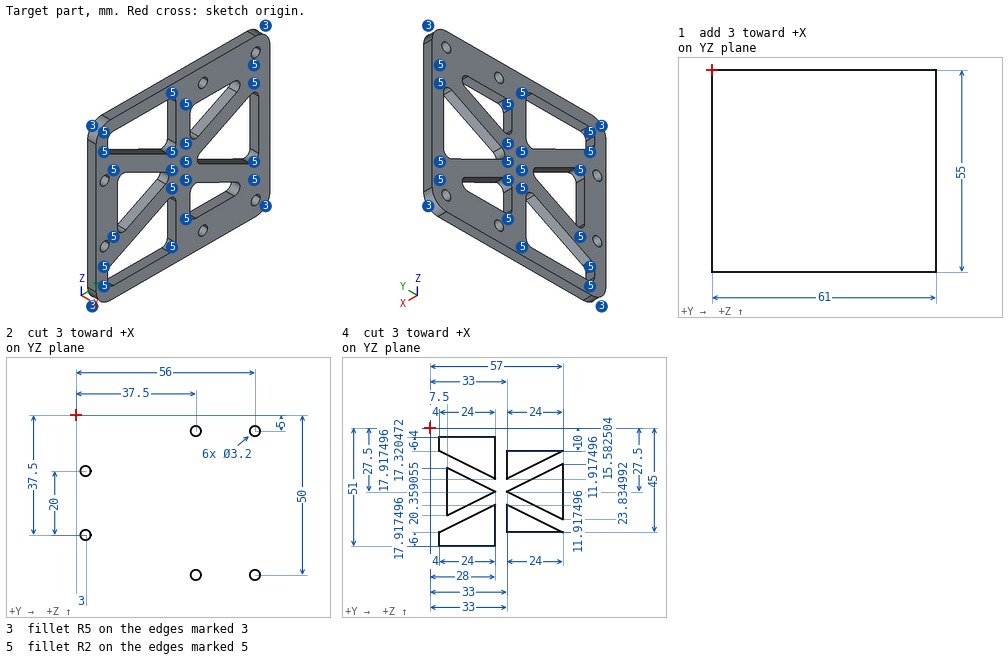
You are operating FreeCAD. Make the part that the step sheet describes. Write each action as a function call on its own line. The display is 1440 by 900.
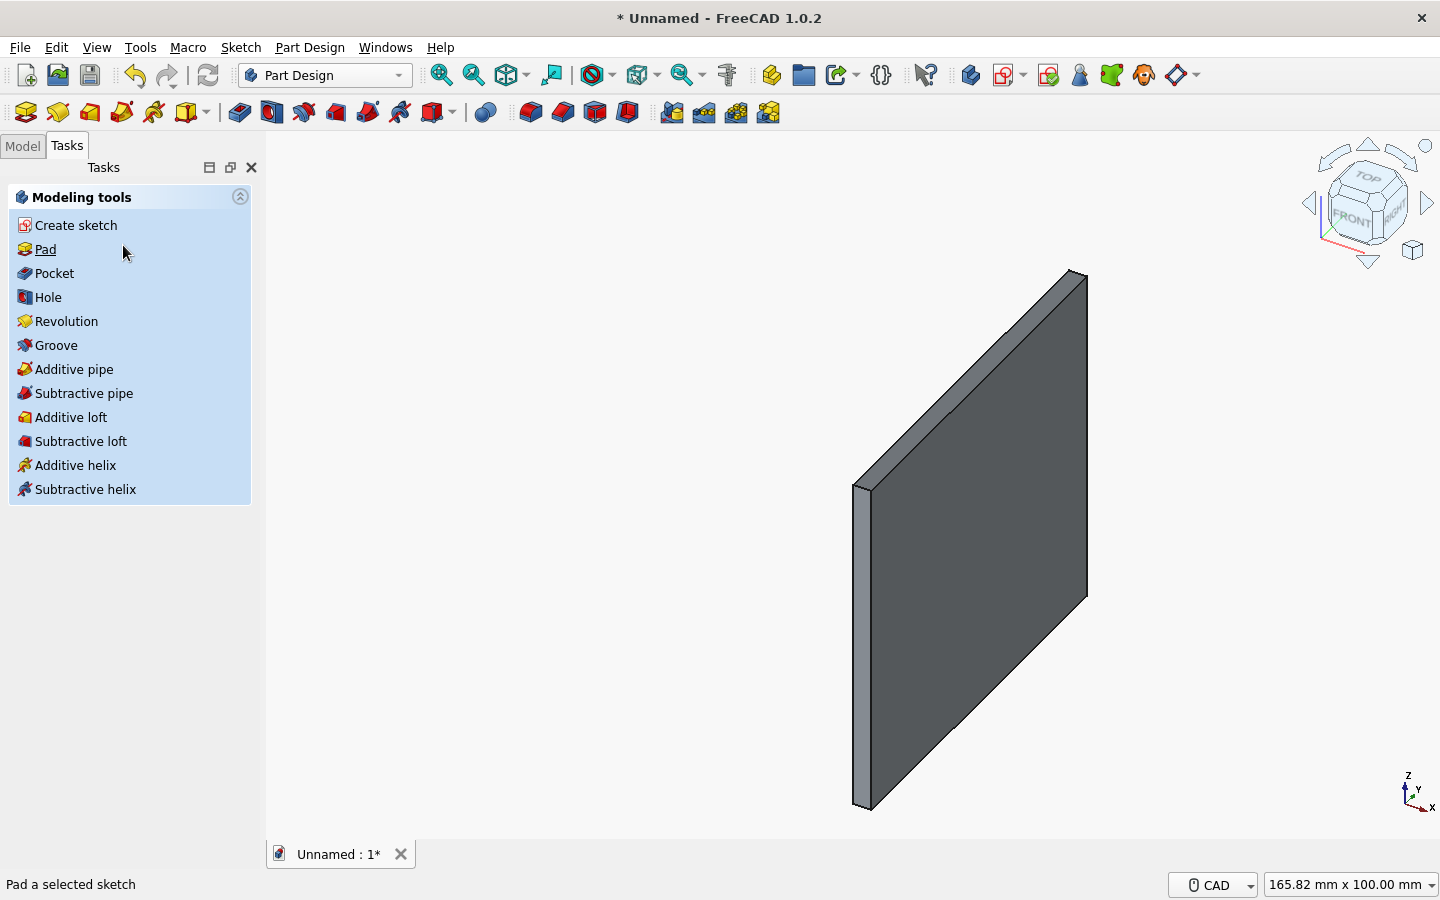
click(240, 112)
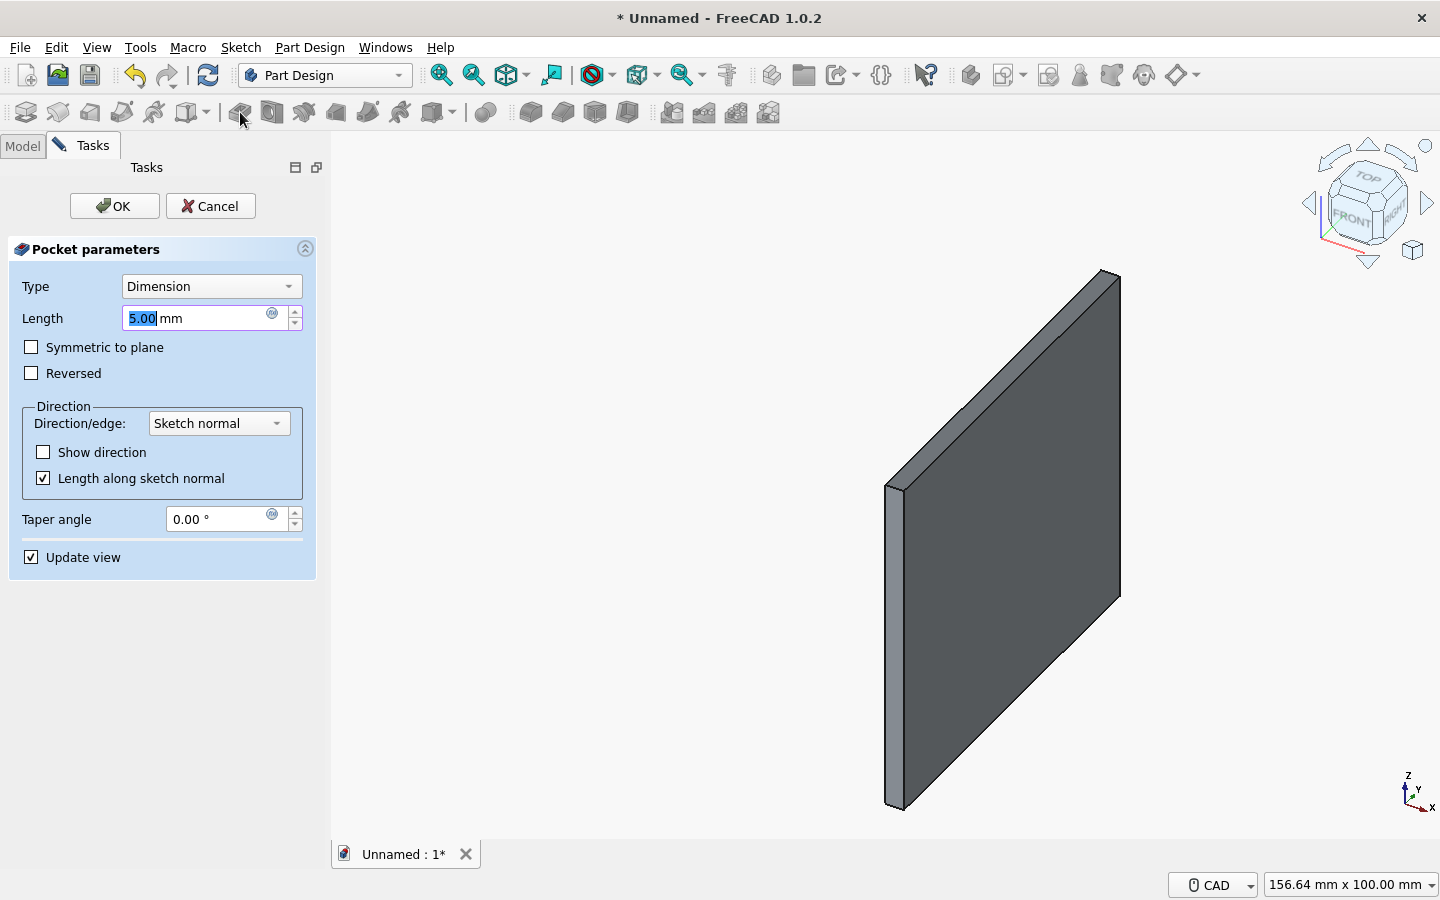
text(3)
key(Tab)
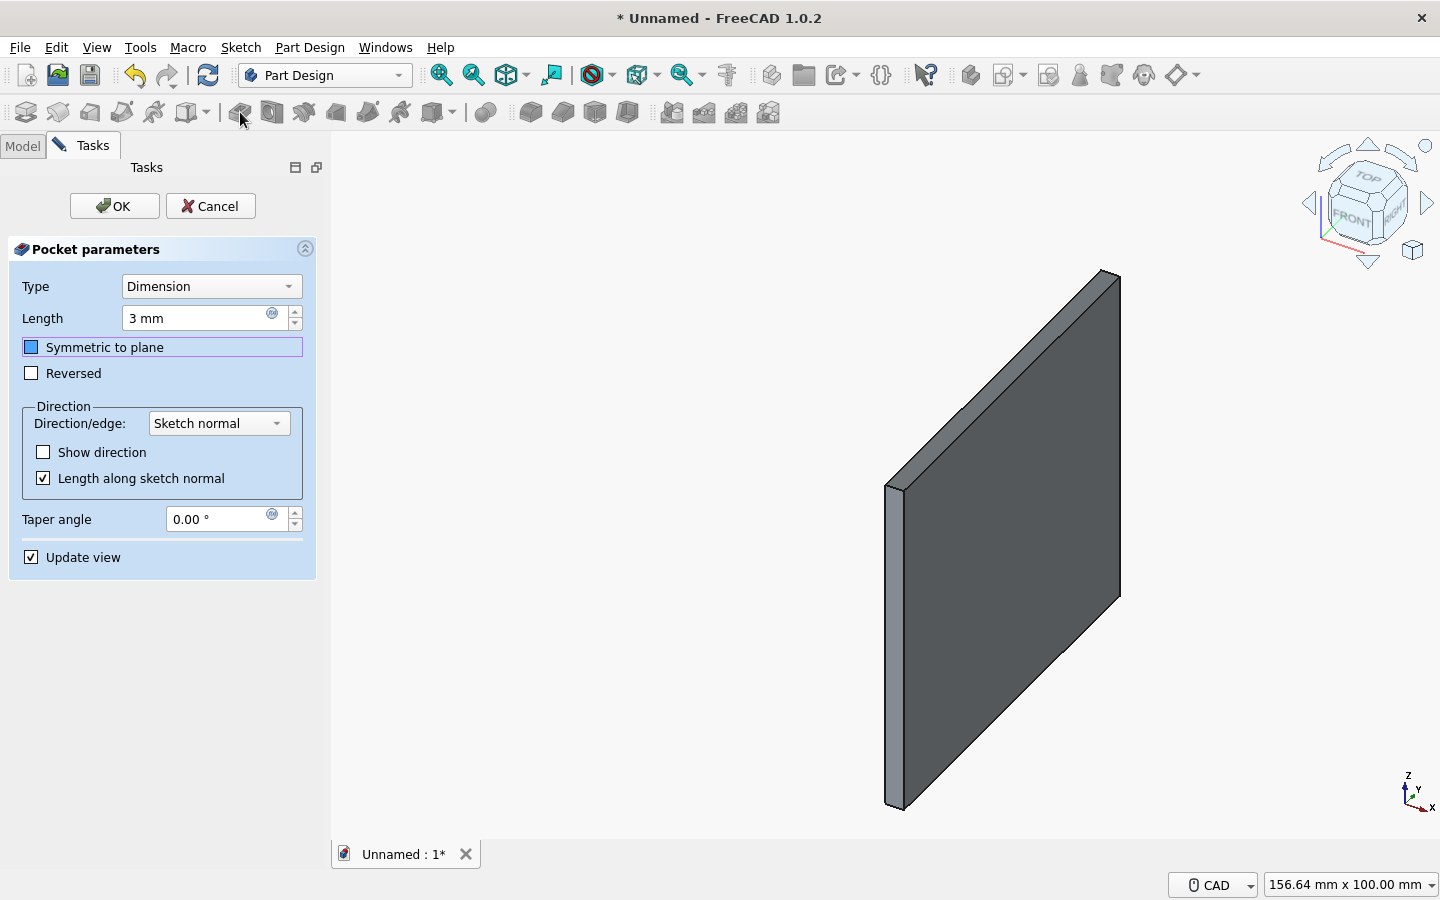
click(30, 373)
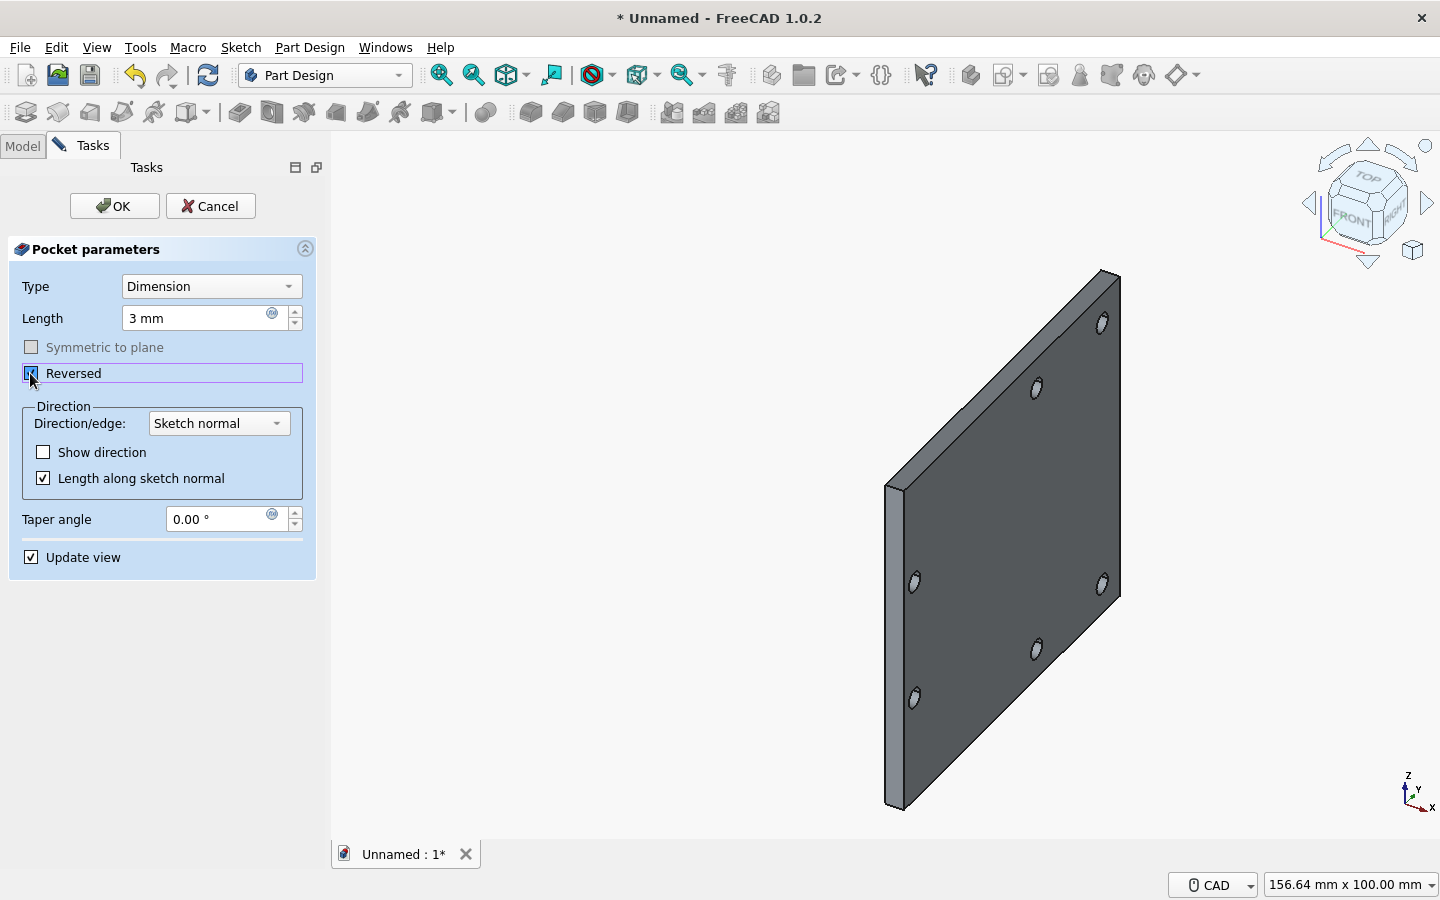
click(115, 206)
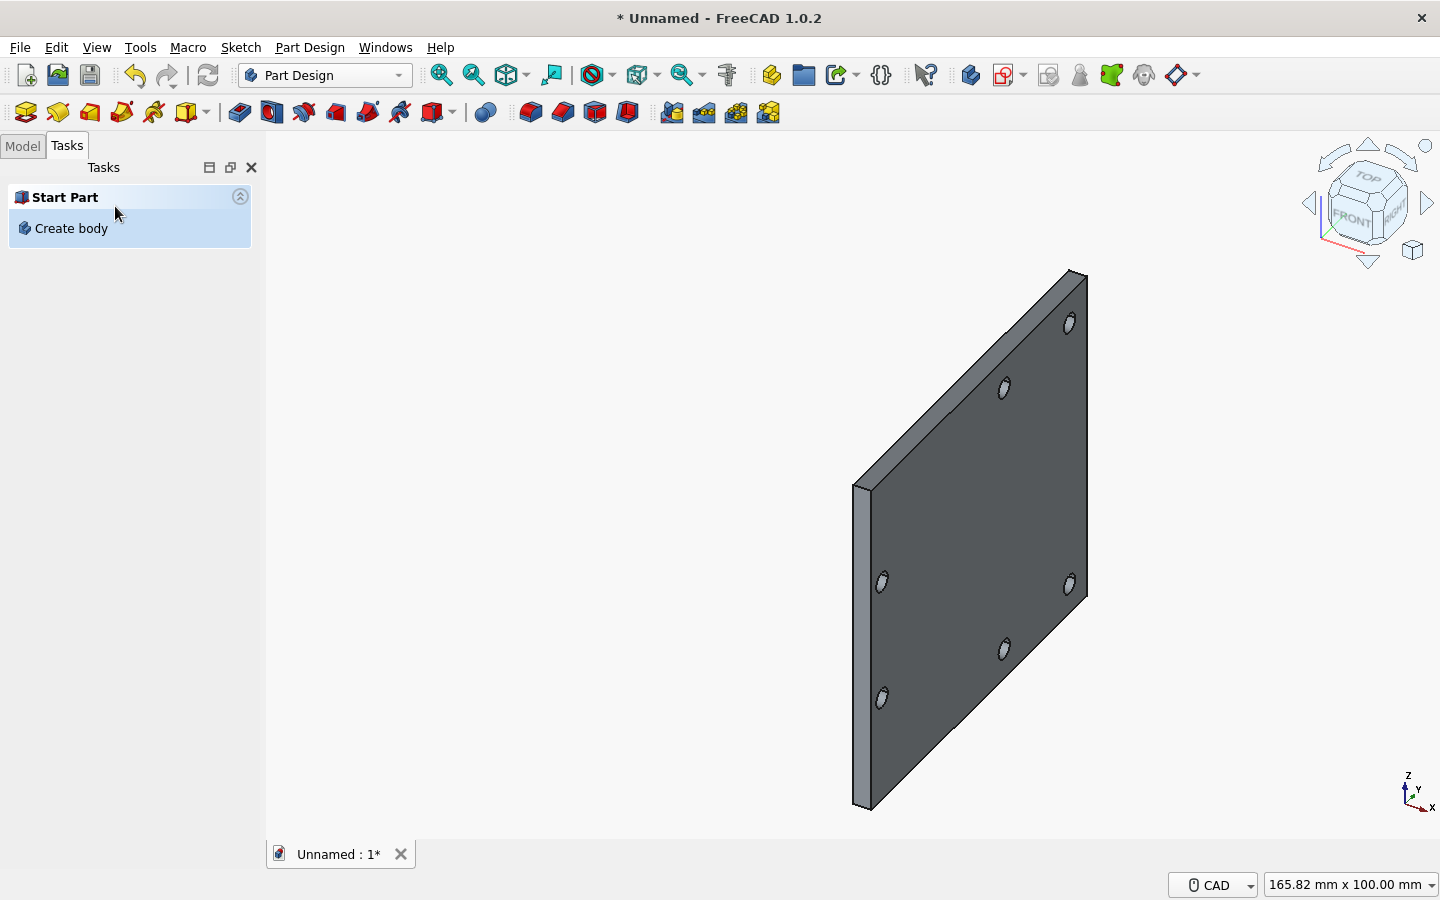
click(862, 487)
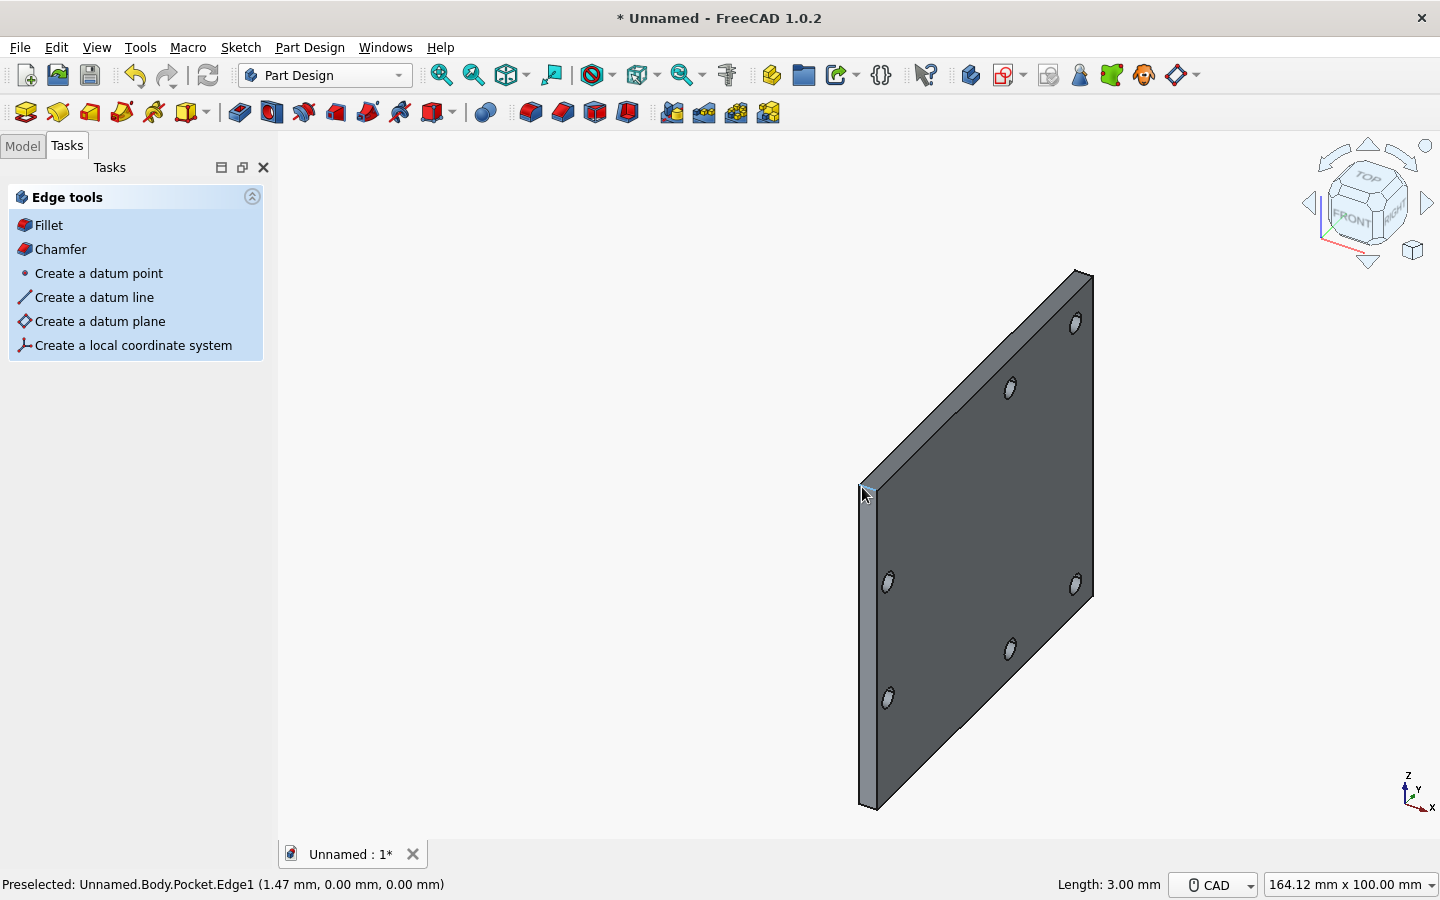
scroll(1084, 273, up, 4)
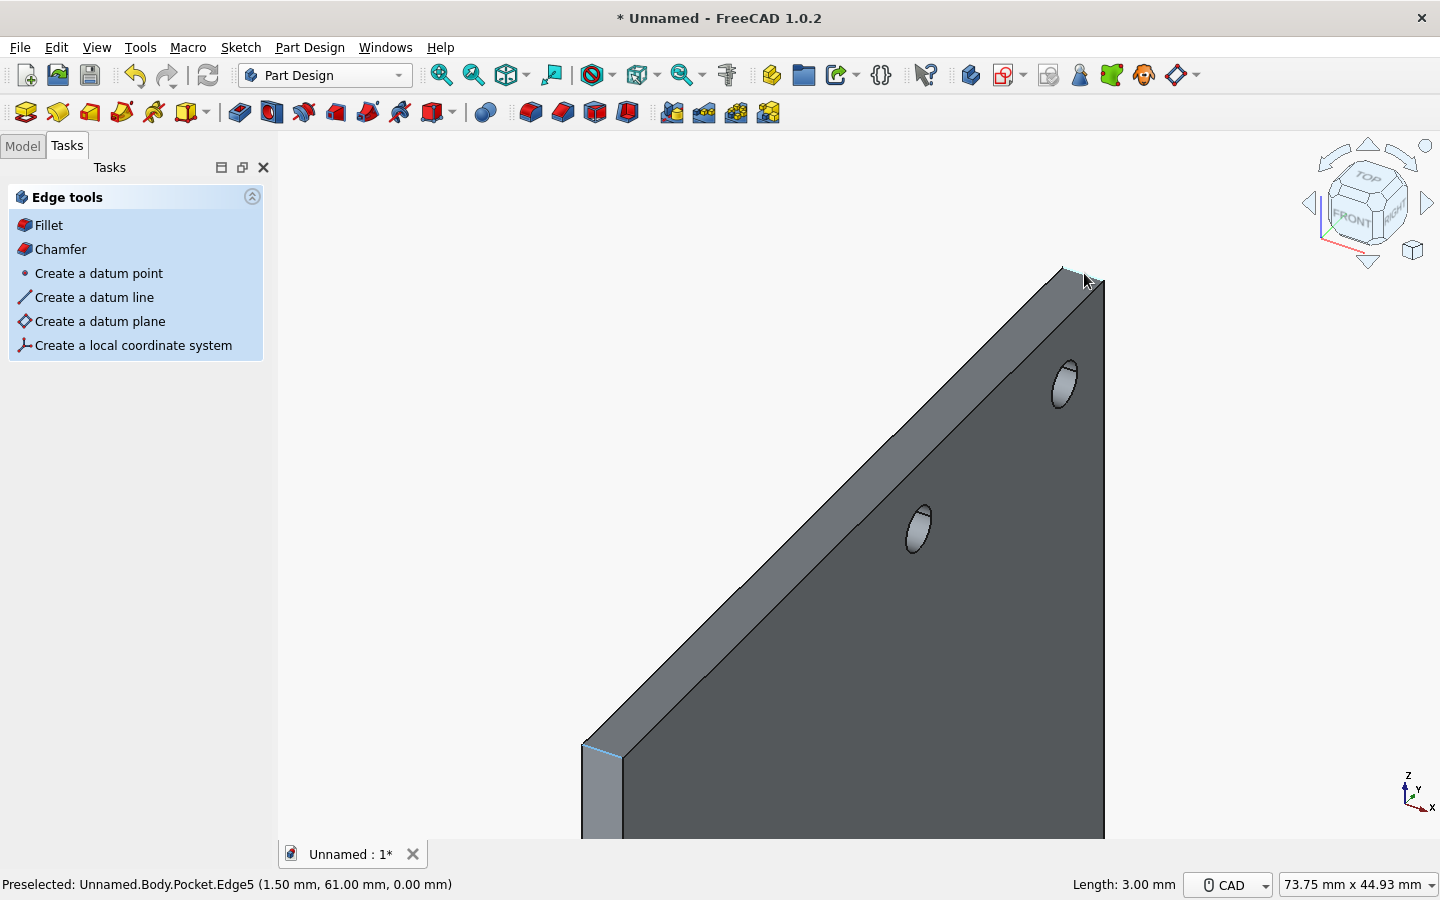
click(442, 76)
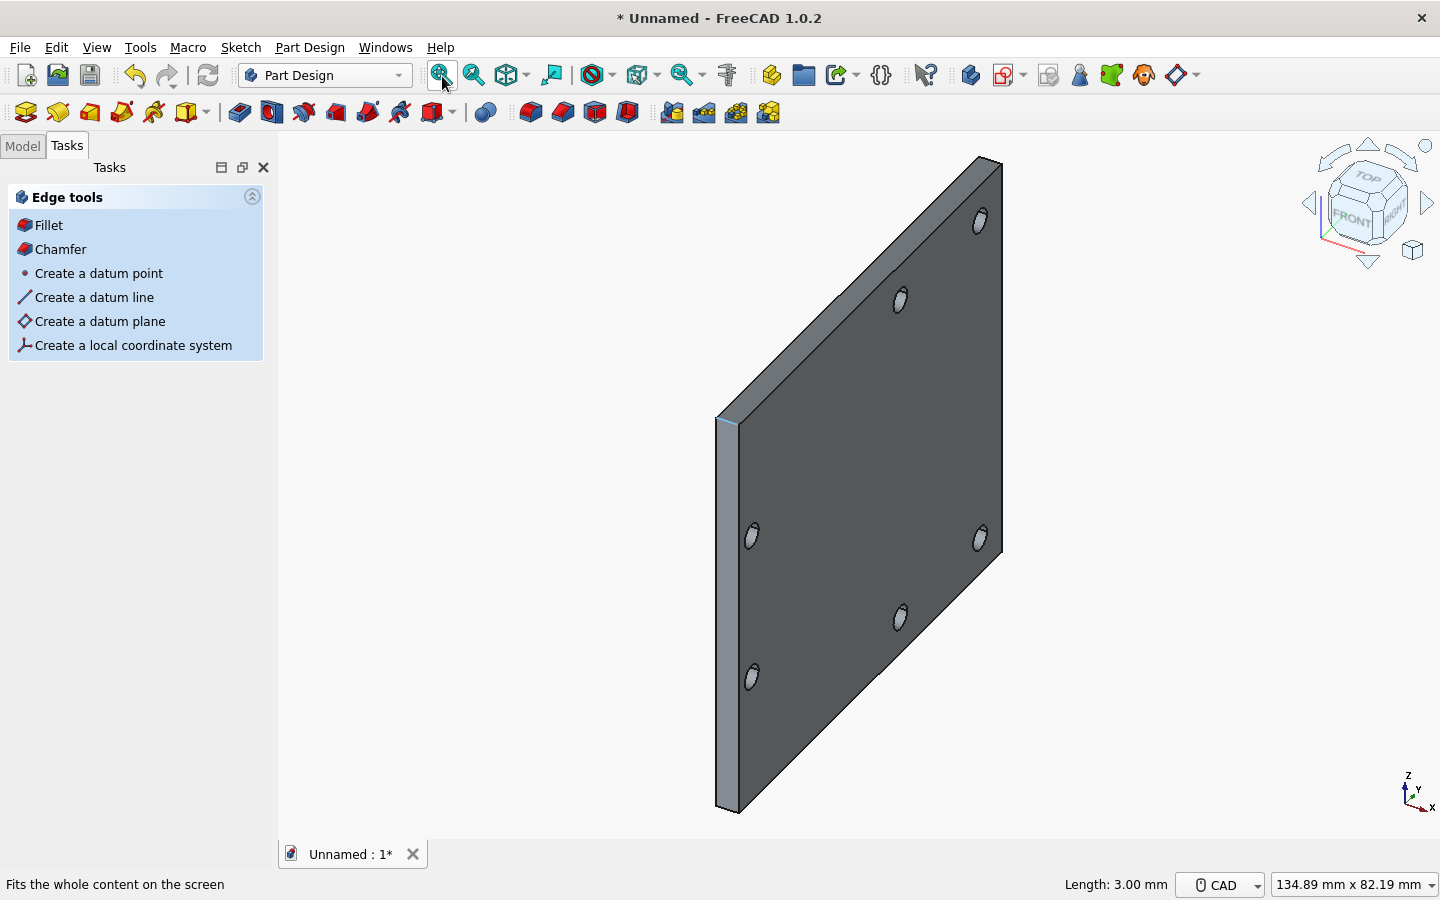
key(0)